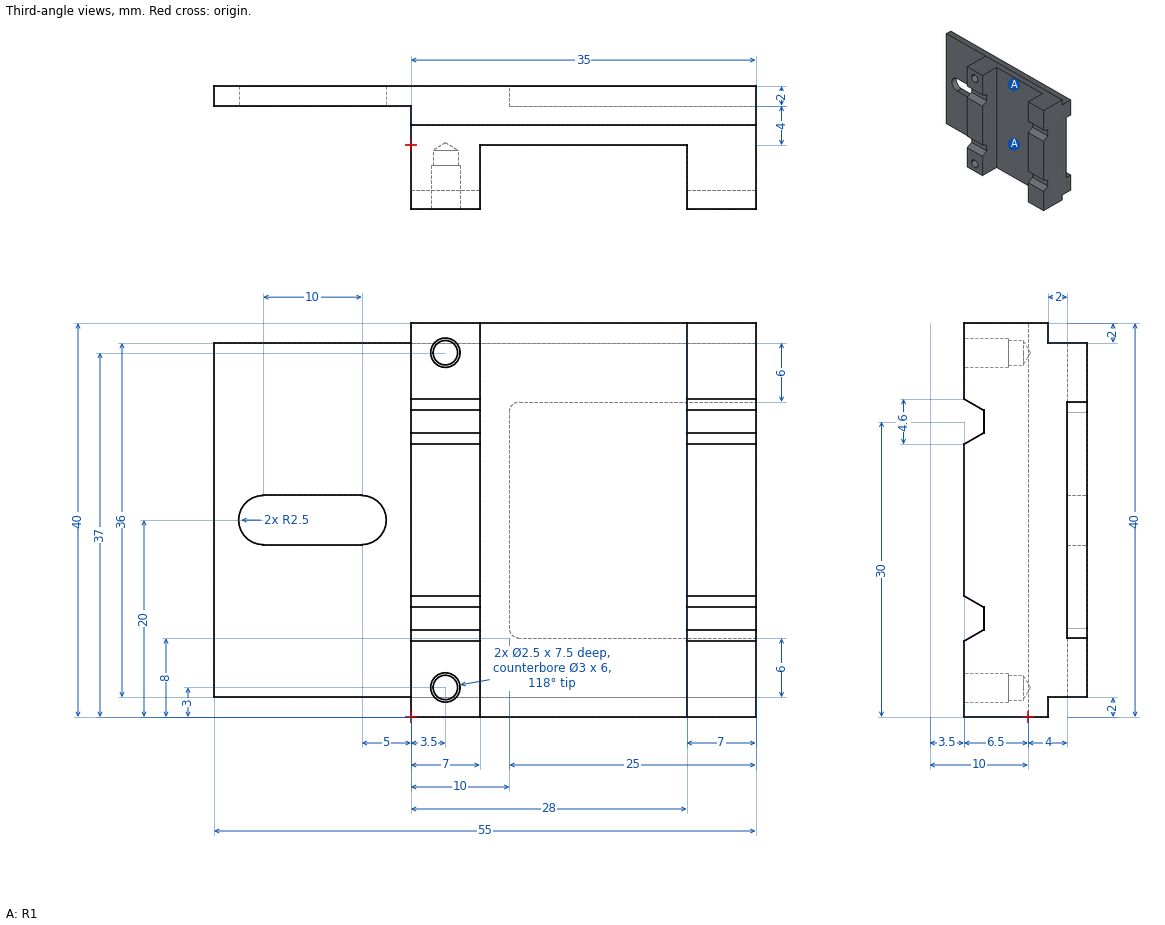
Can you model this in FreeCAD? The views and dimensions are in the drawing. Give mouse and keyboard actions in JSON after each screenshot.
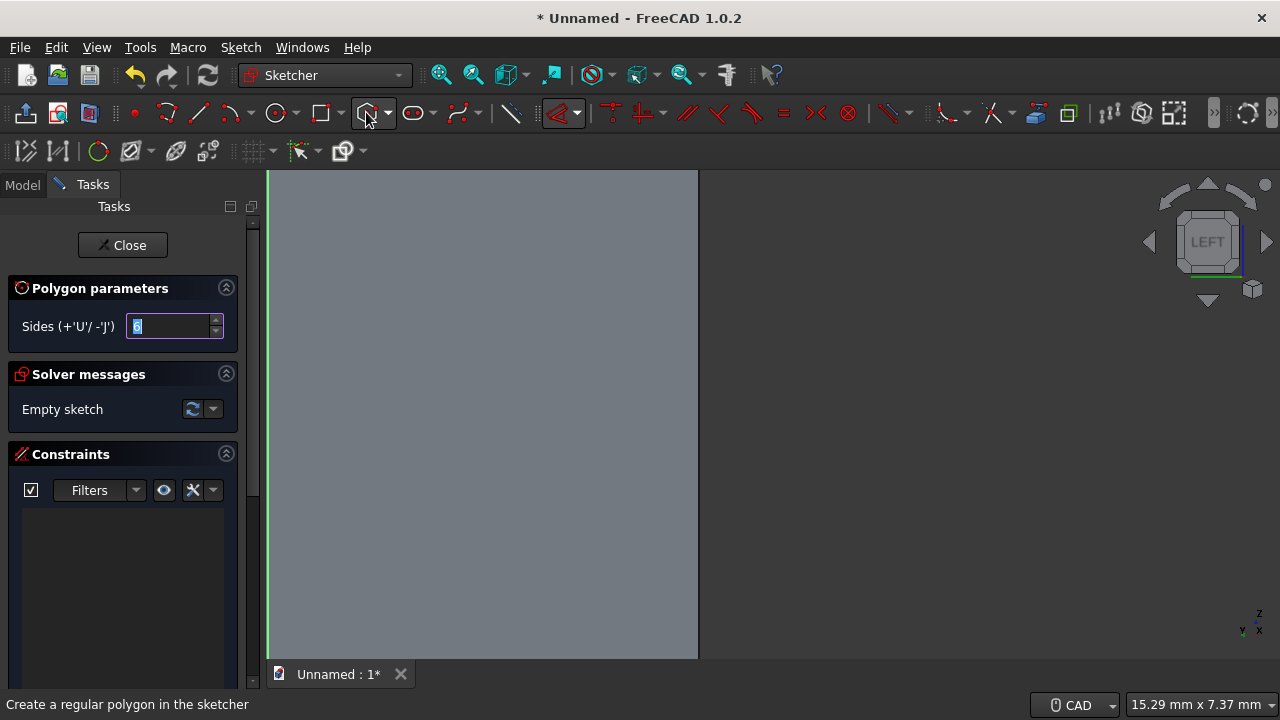
{"action": "left_click", "coordinate": [699, 409]}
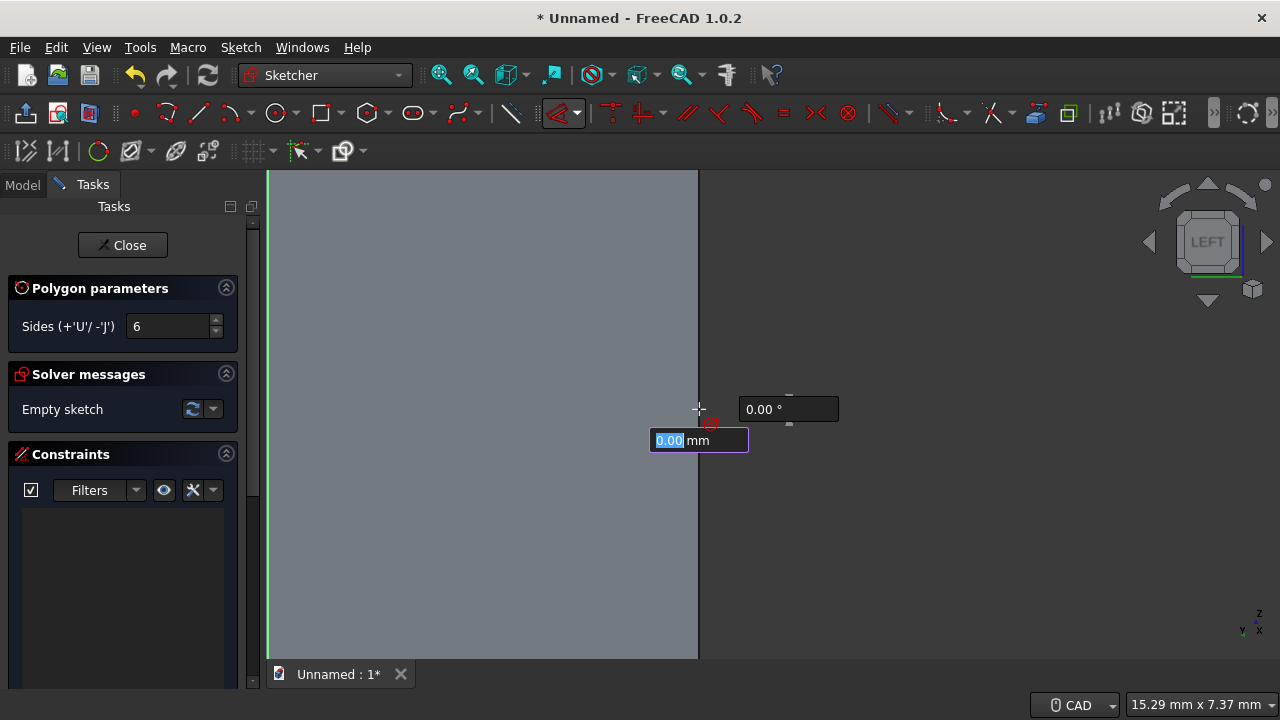
{"action": "left_click", "coordinate": [699, 562]}
{"action": "key", "text": "Escape"}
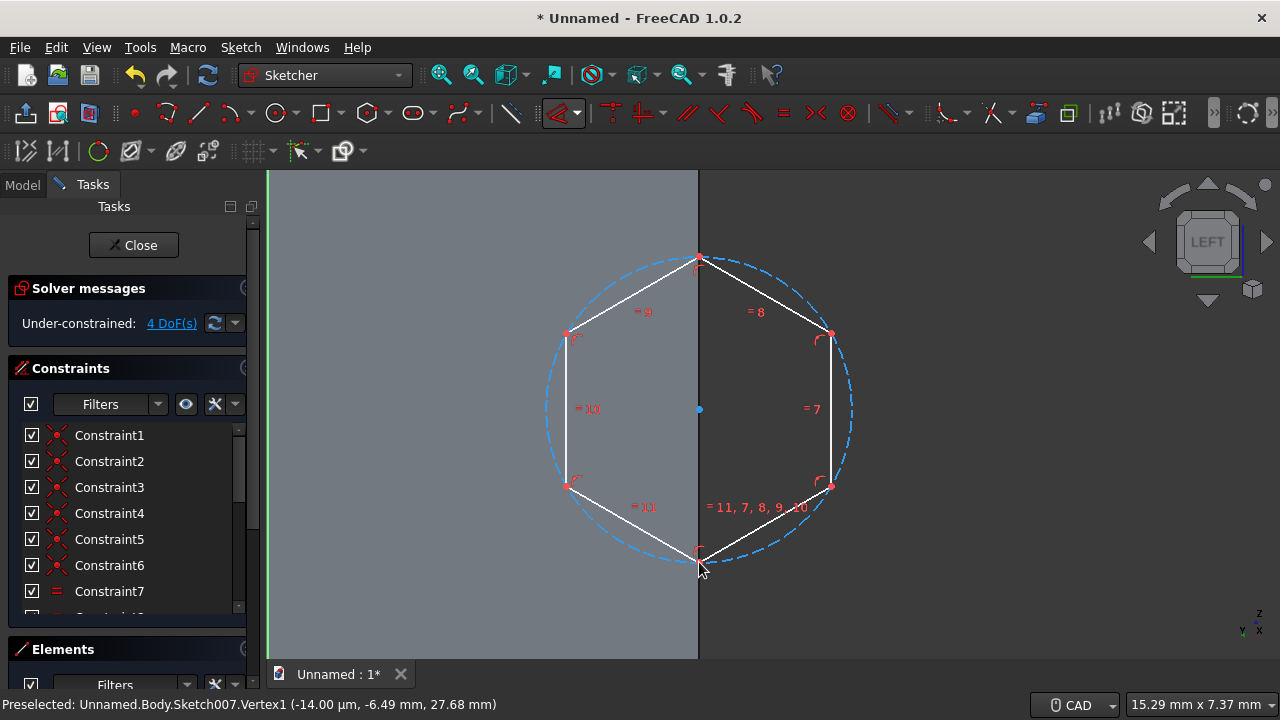
{"action": "left_click", "coordinate": [832, 441]}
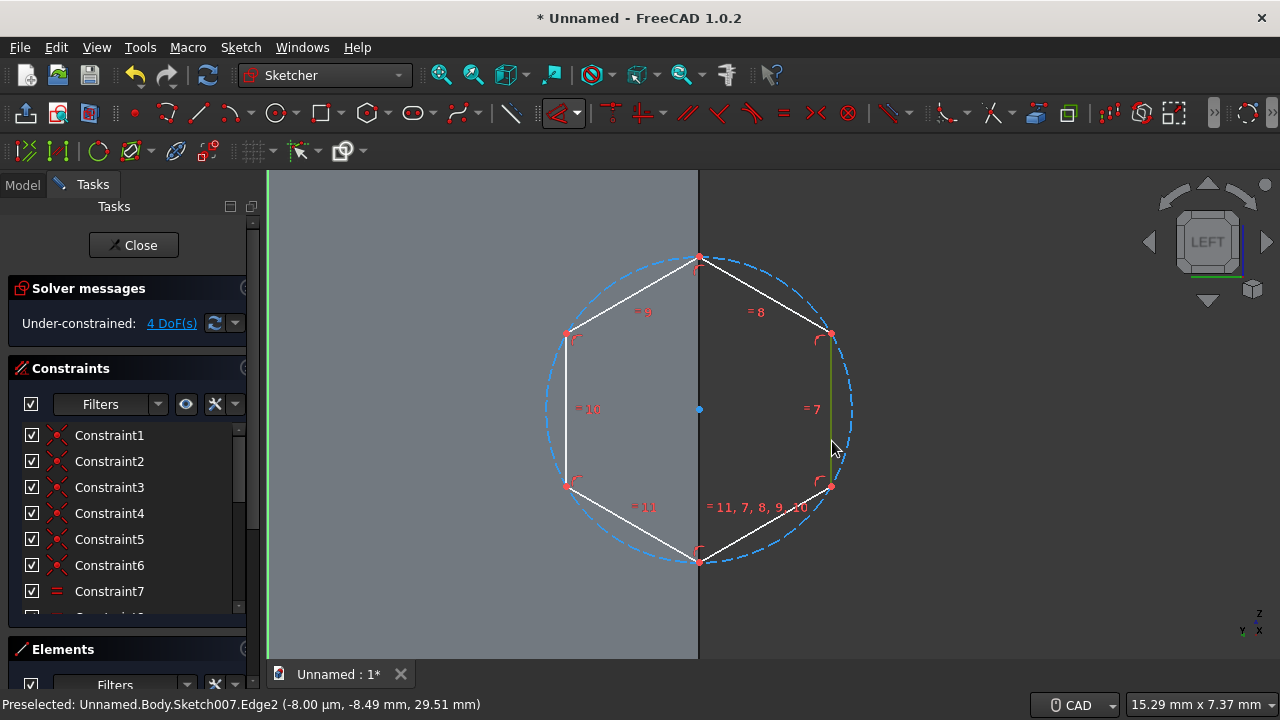
{"action": "key", "text": "v"}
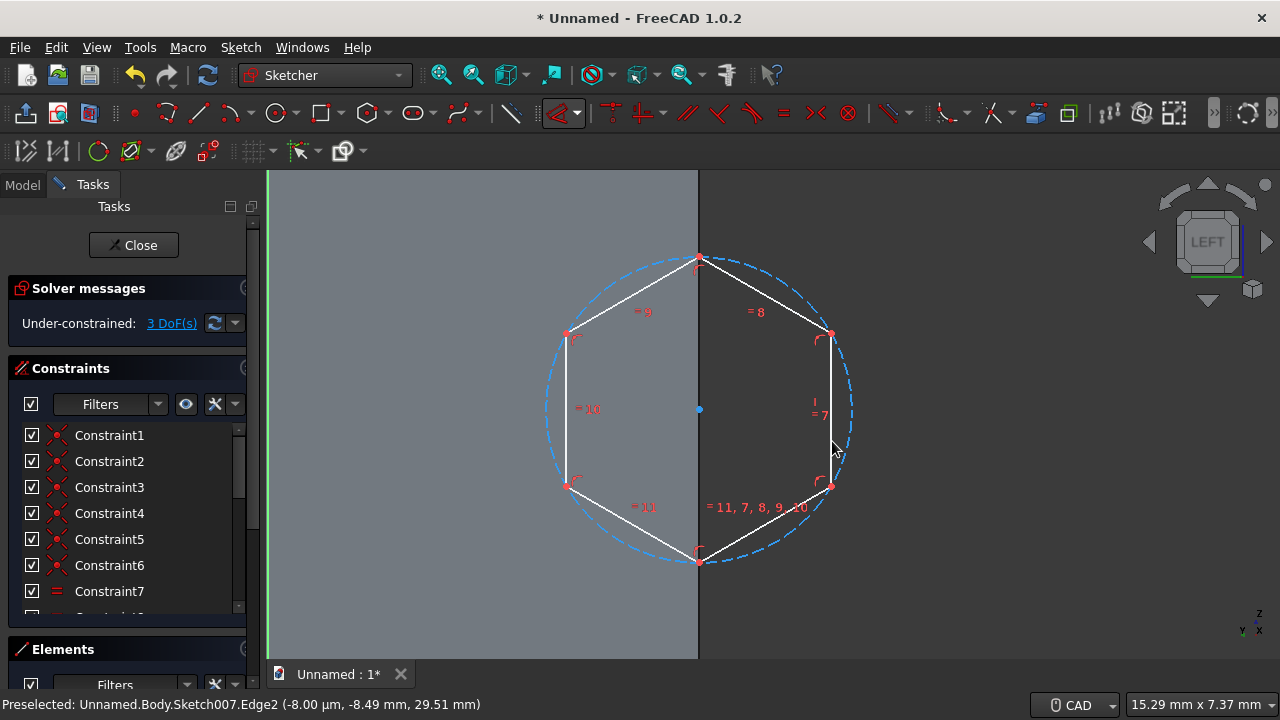
{"action": "left_click", "coordinate": [699, 563]}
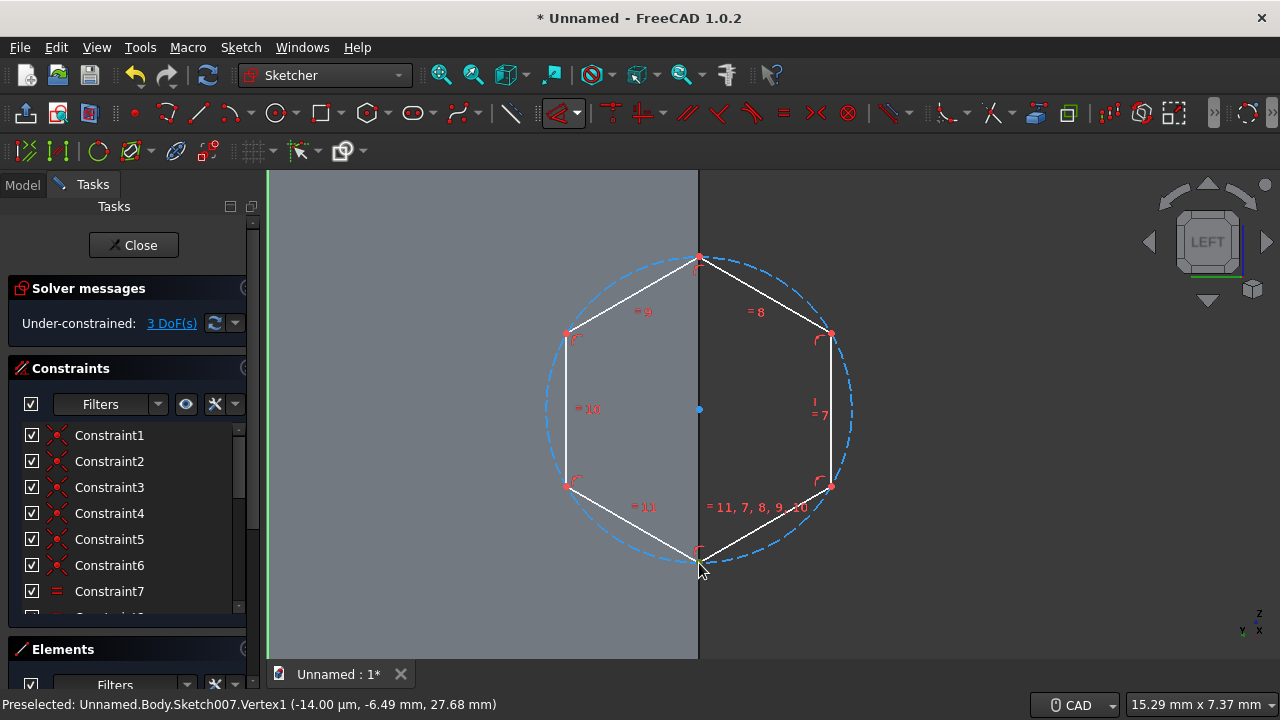
{"action": "left_click", "coordinate": [699, 257]}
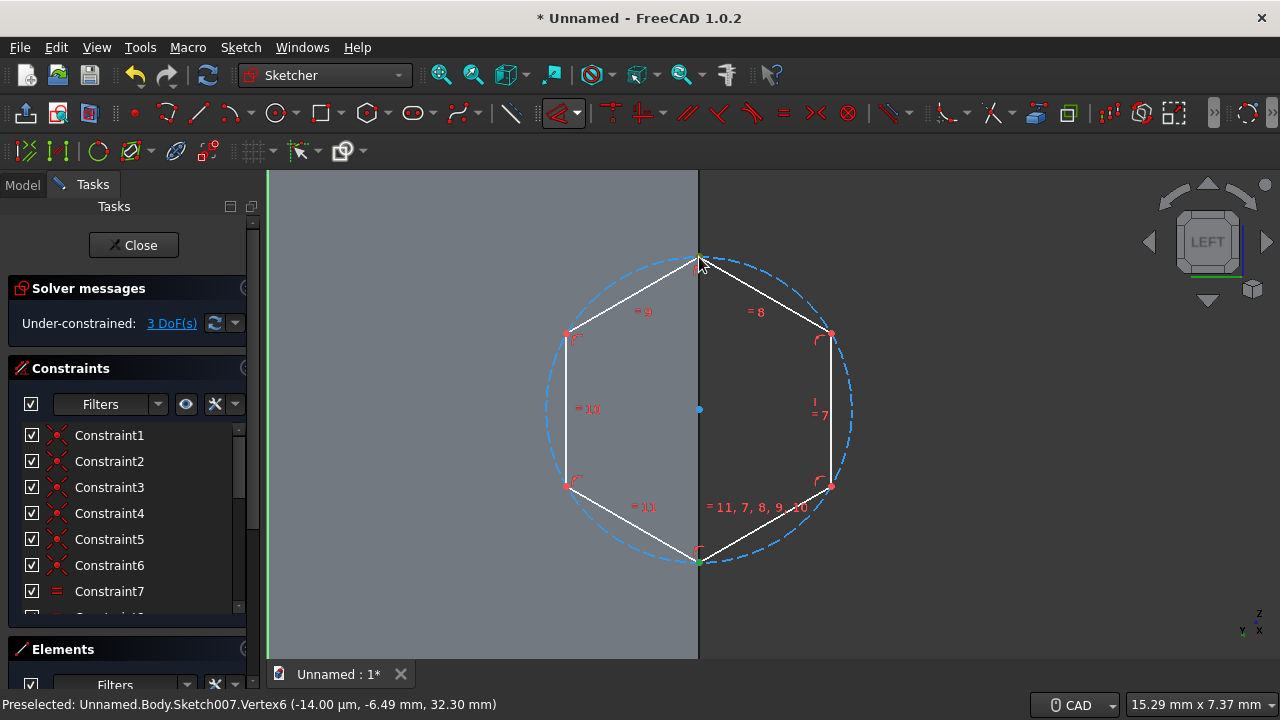
{"action": "left_click", "coordinate": [580, 114]}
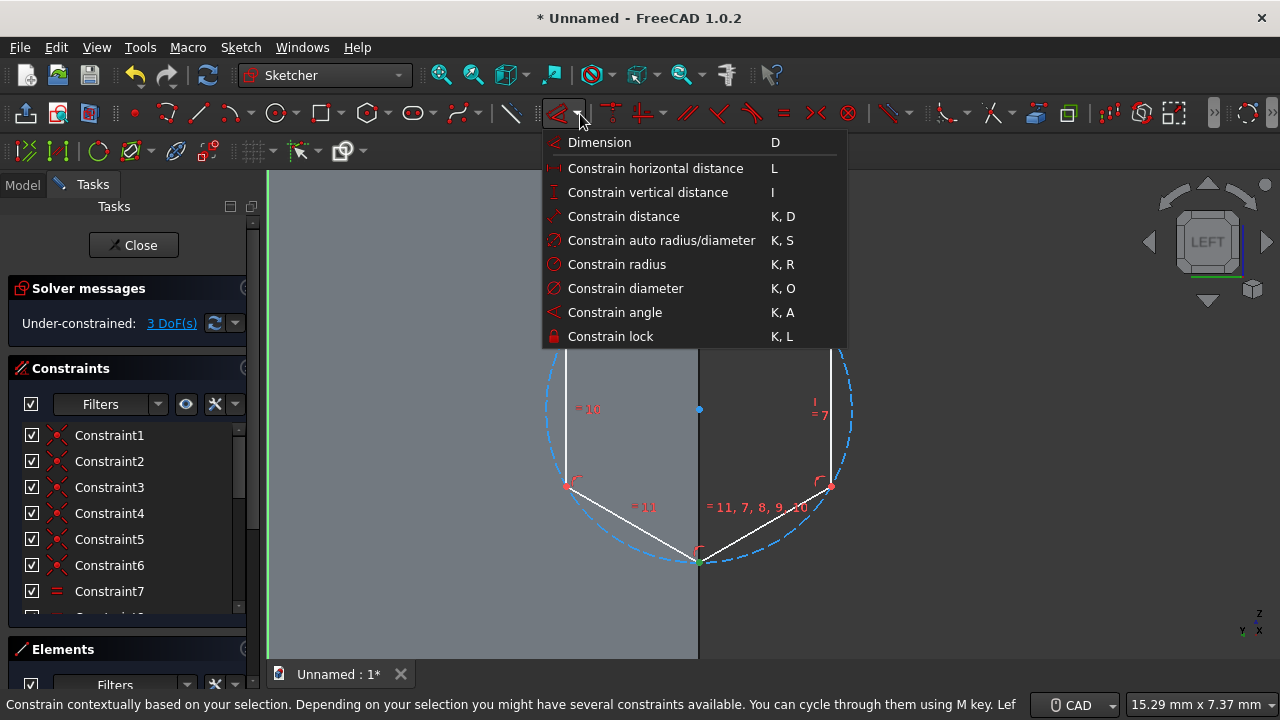
{"action": "left_click", "coordinate": [695, 192]}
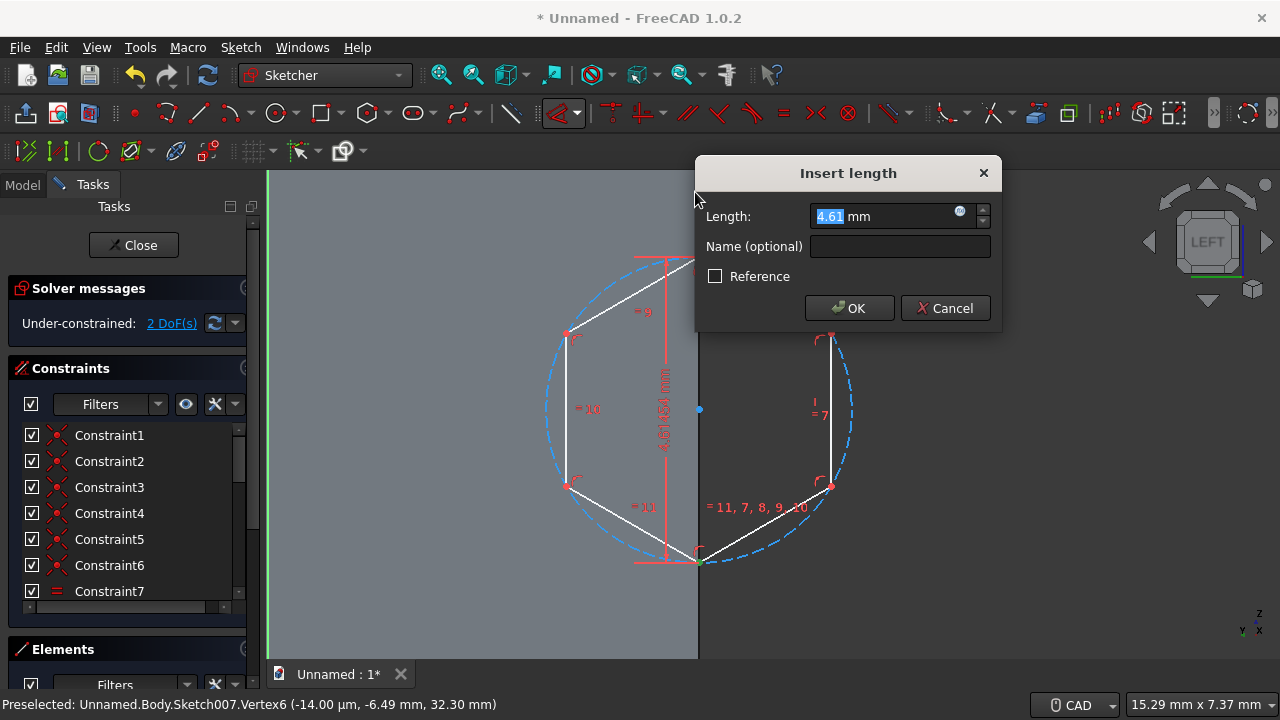
{"action": "type", "text": "4.6"}
{"action": "key", "text": "Return"}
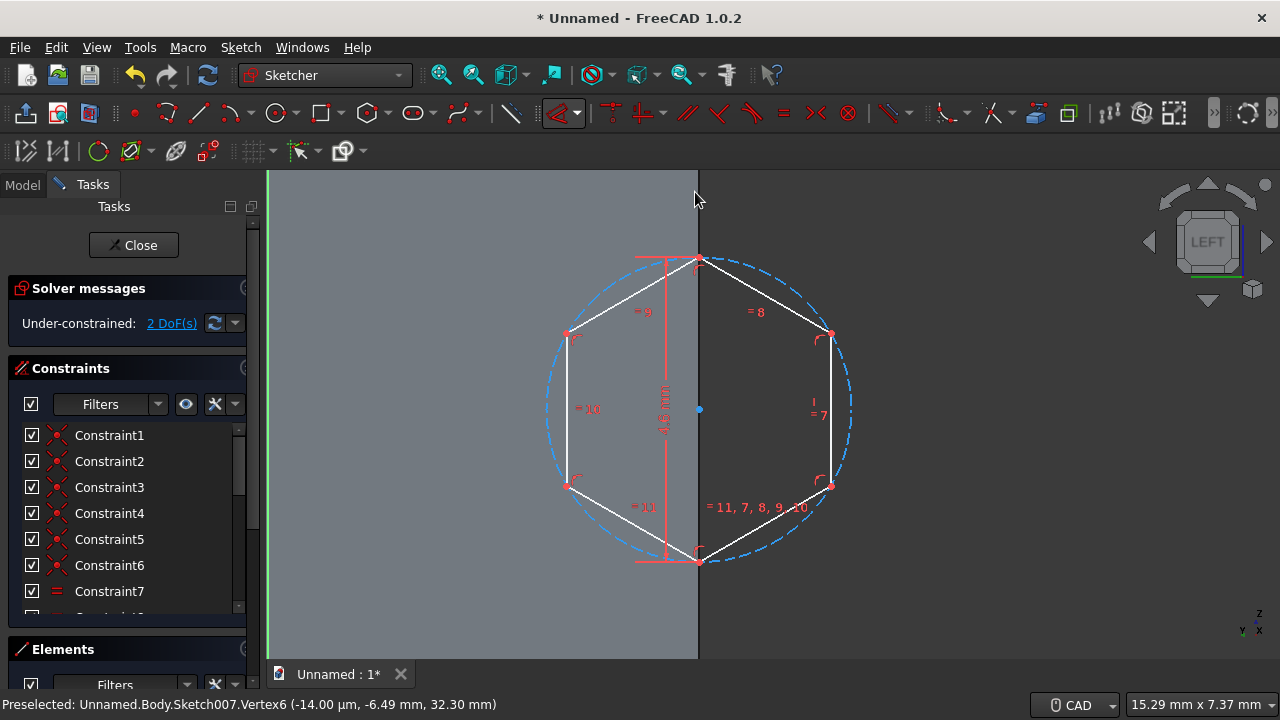
{"action": "left_click", "coordinate": [699, 410]}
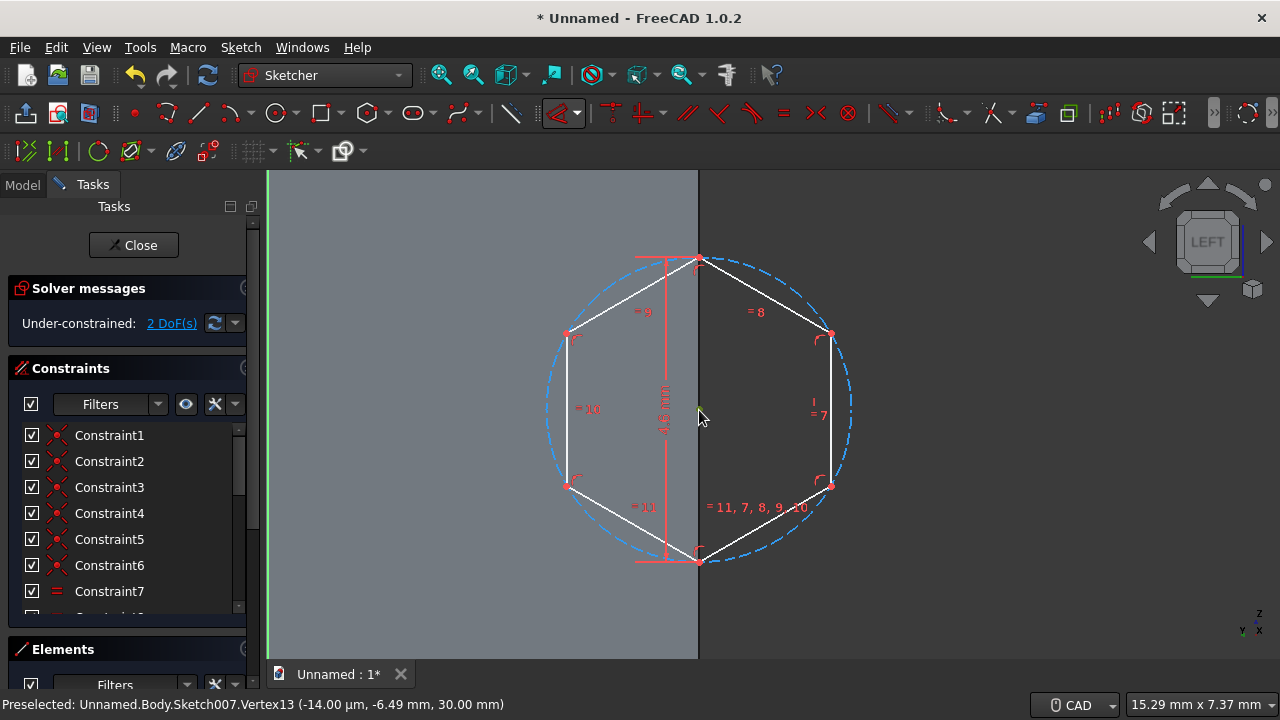
{"action": "key", "text": "i"}